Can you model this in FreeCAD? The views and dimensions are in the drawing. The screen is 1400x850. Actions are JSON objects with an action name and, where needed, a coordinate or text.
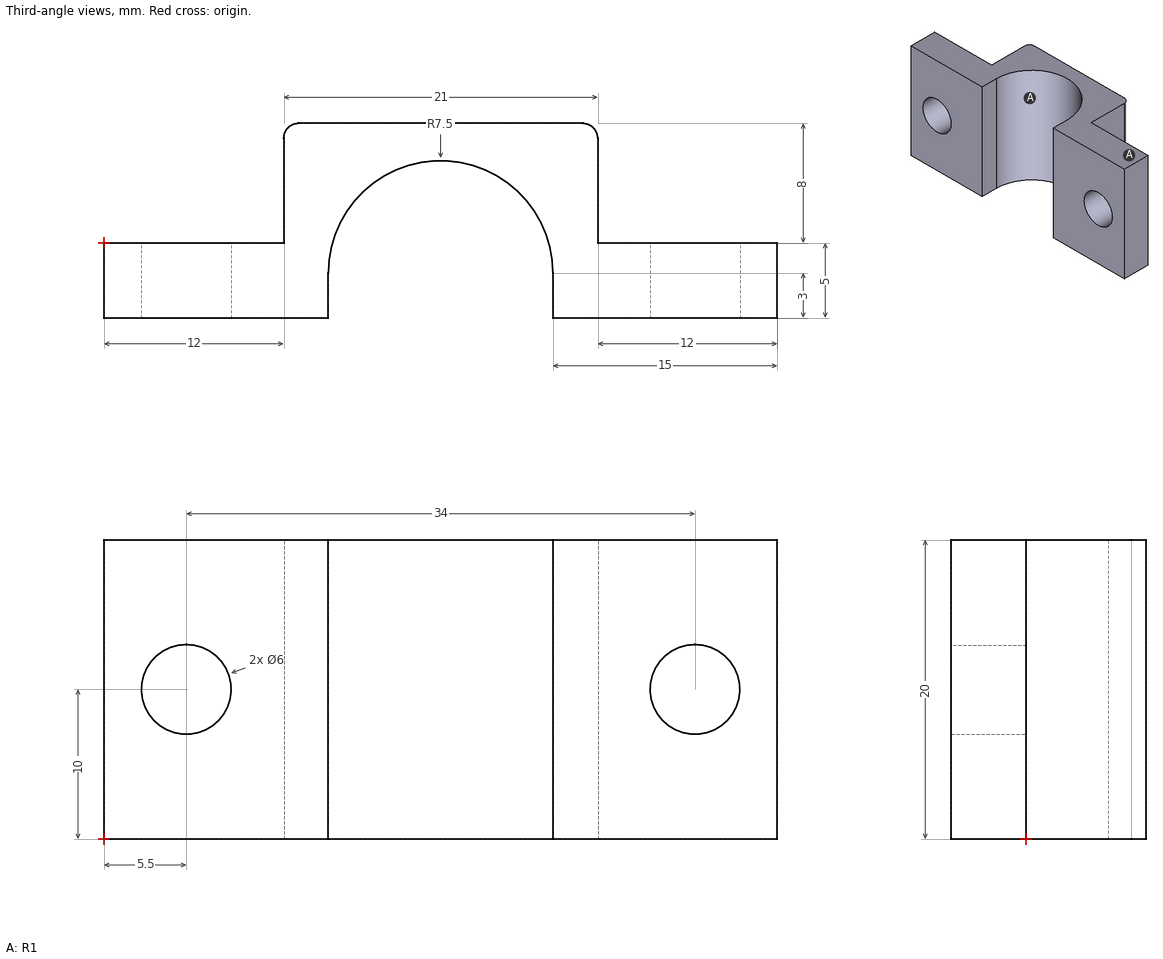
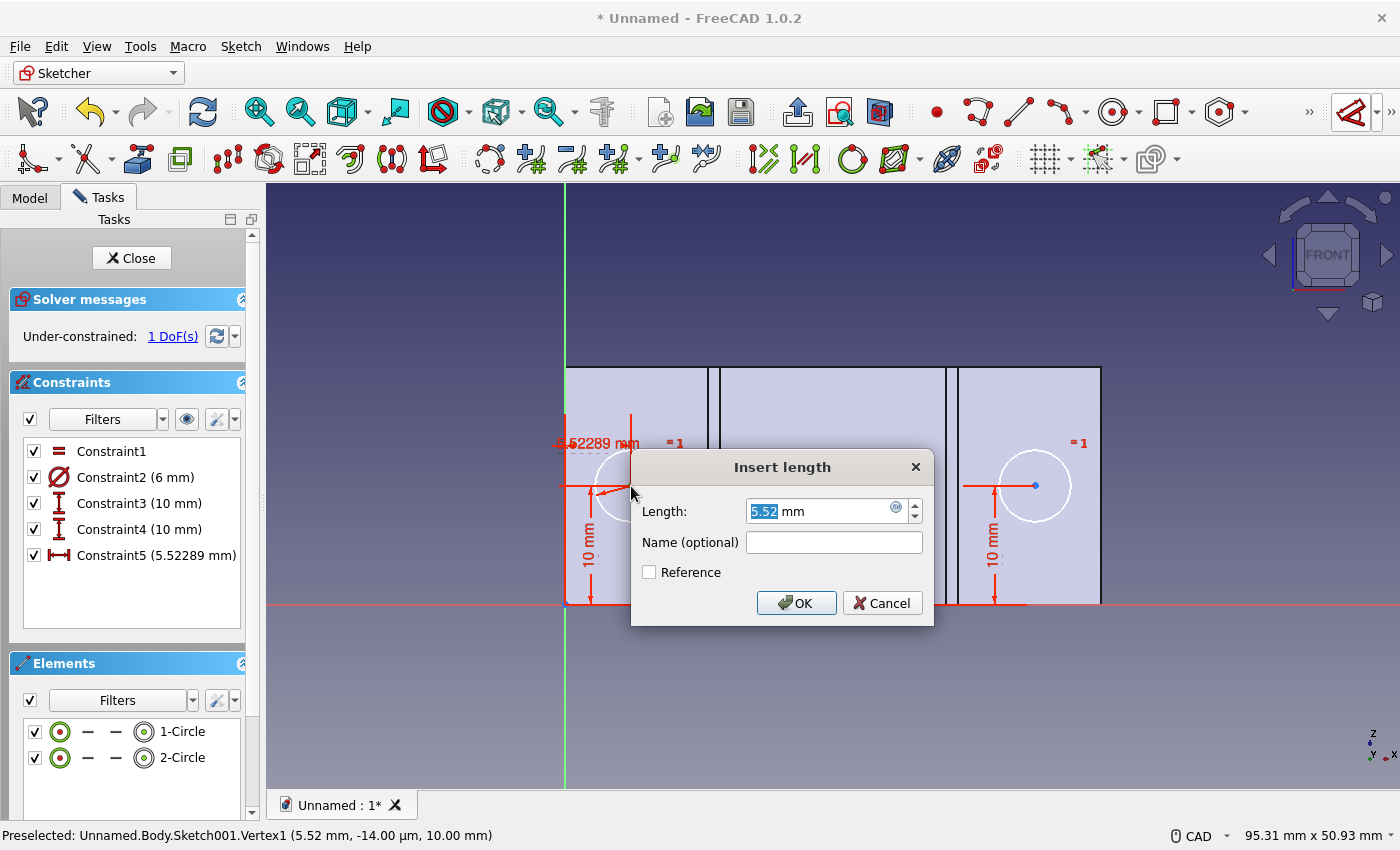
{"action": "type", "text": "5.5"}
{"action": "key", "text": "Return"}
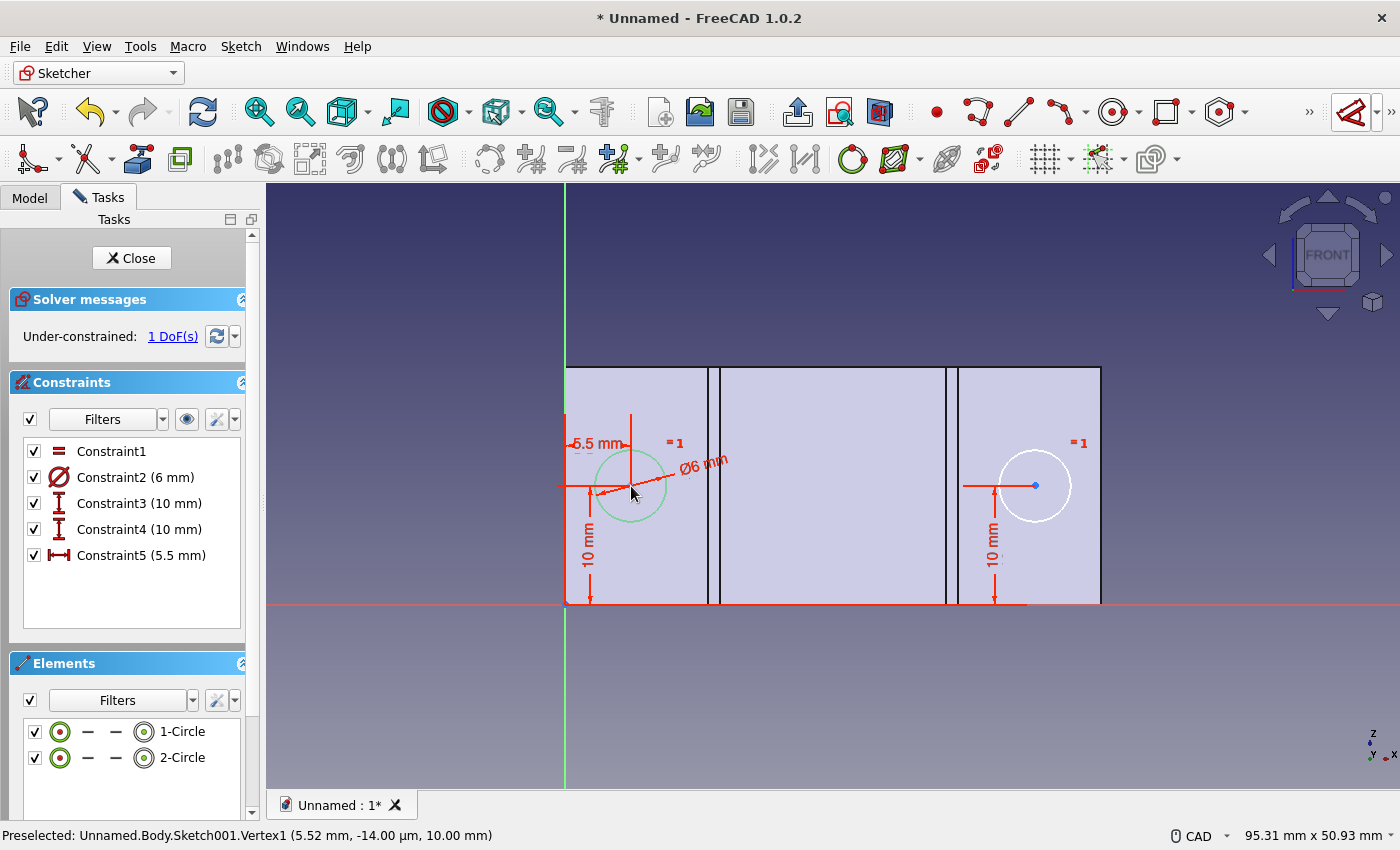
{"action": "left_click", "coordinate": [631, 486]}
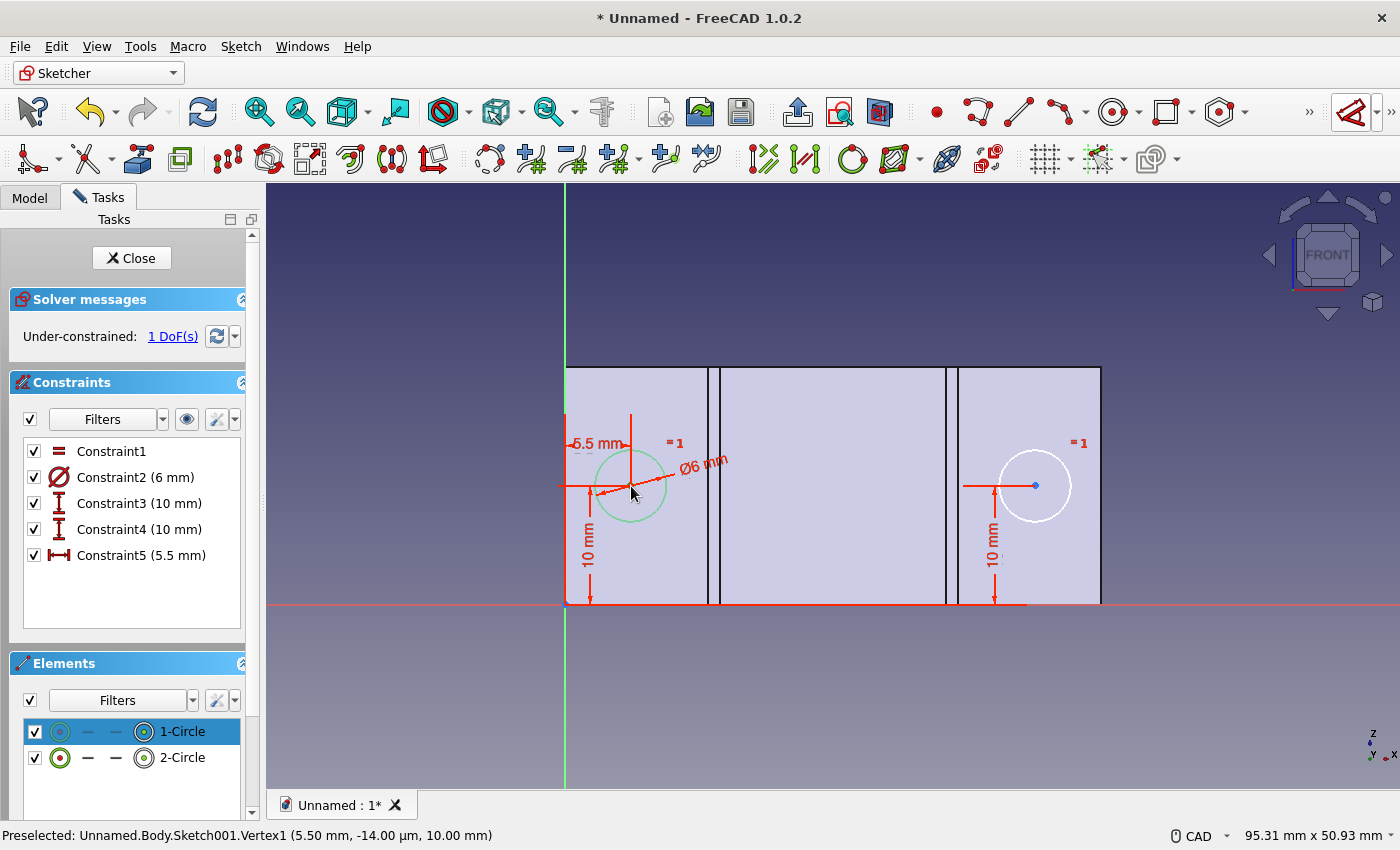
{"action": "left_click", "coordinate": [1035, 486]}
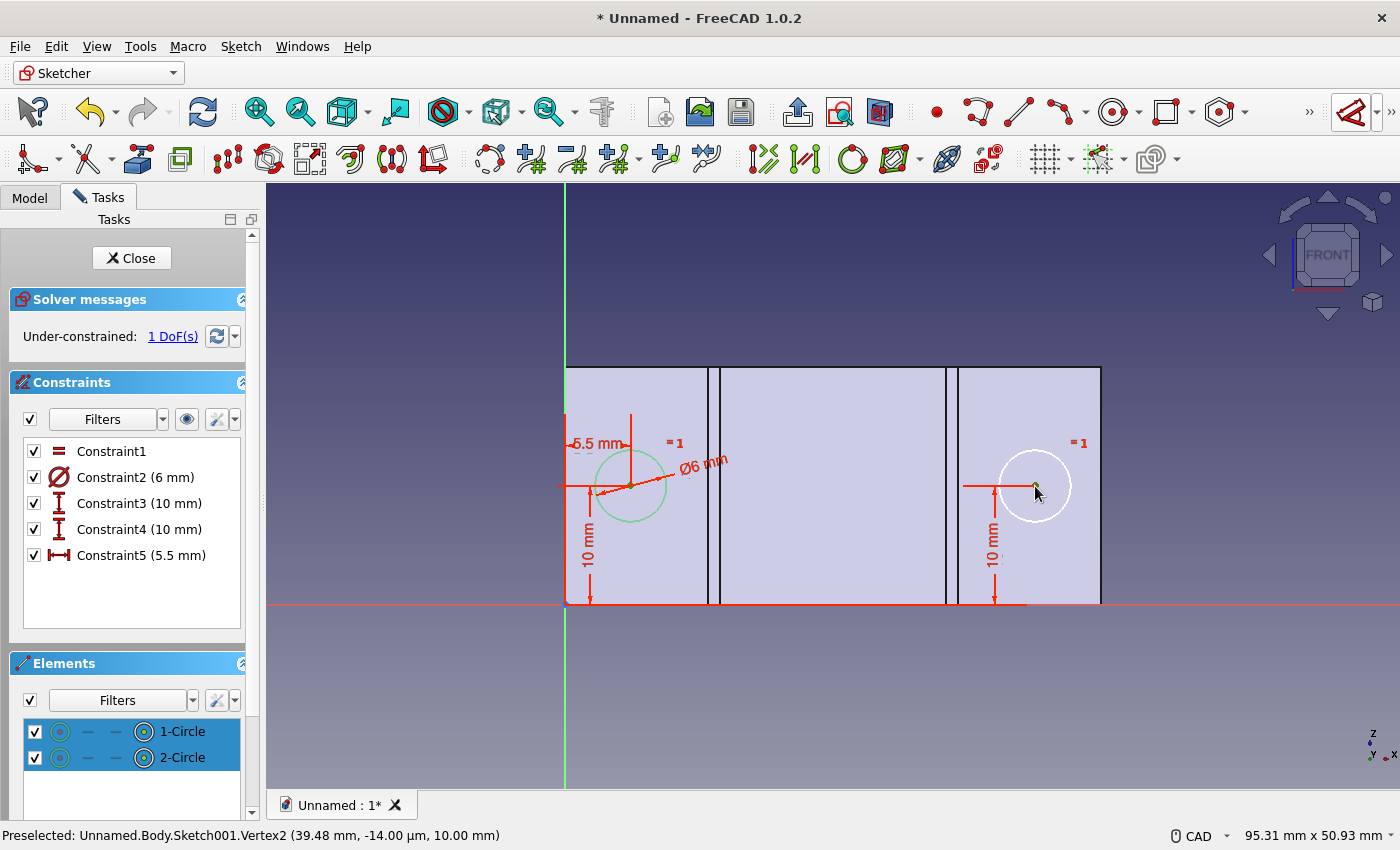
{"action": "key", "text": "l"}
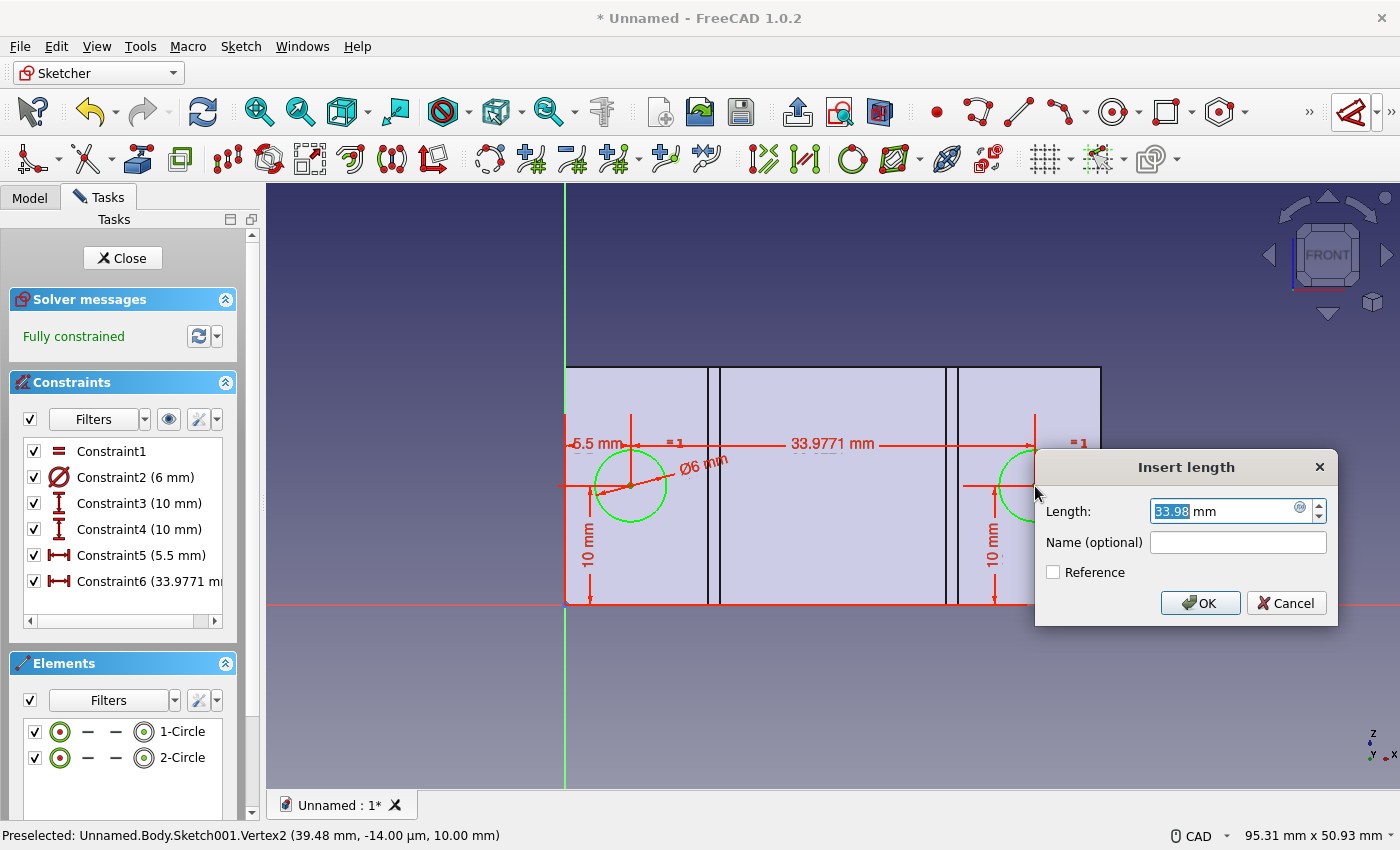
{"action": "type", "text": "34"}
{"action": "key", "text": "Return"}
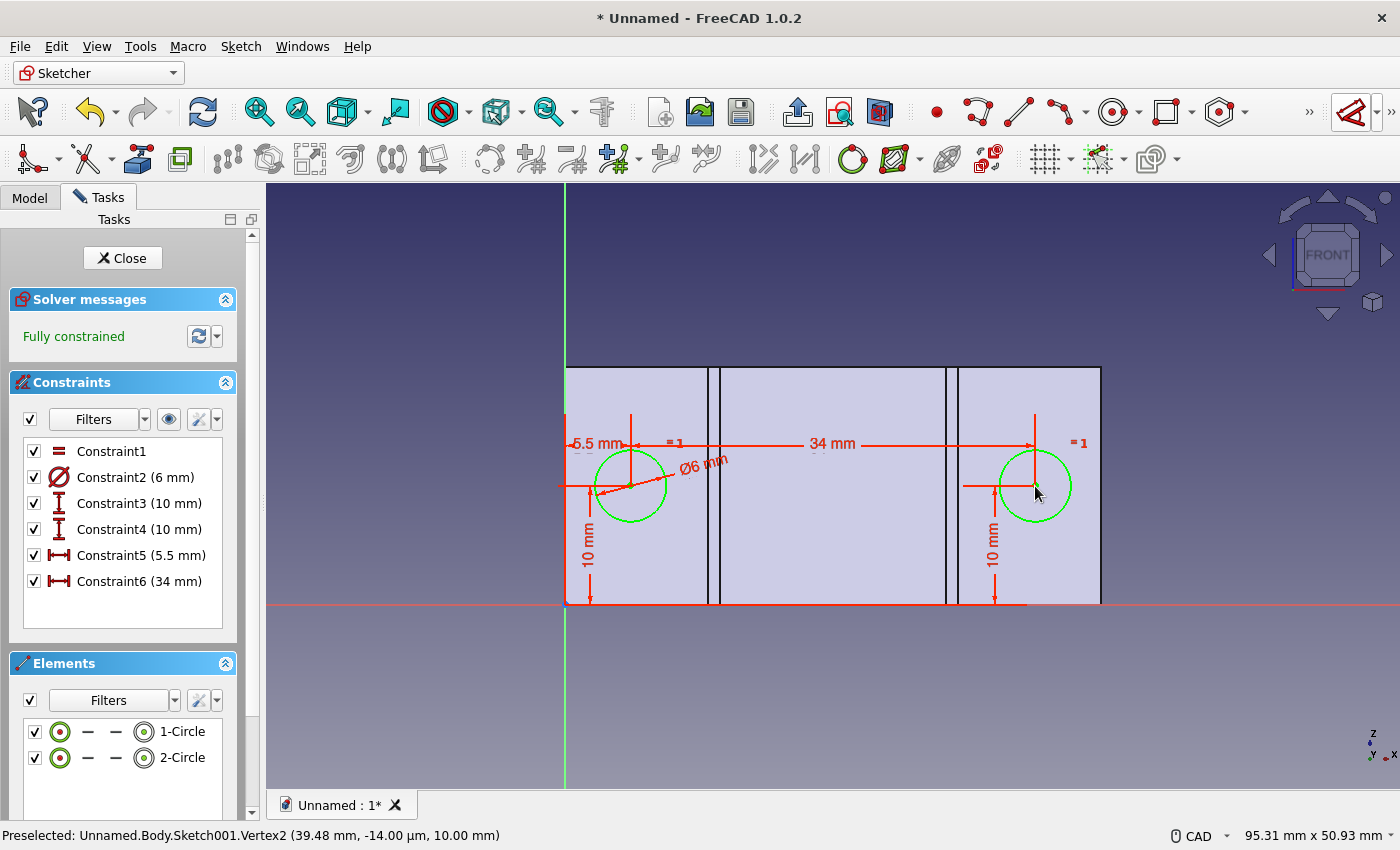
{"action": "left_click", "coordinate": [123, 258]}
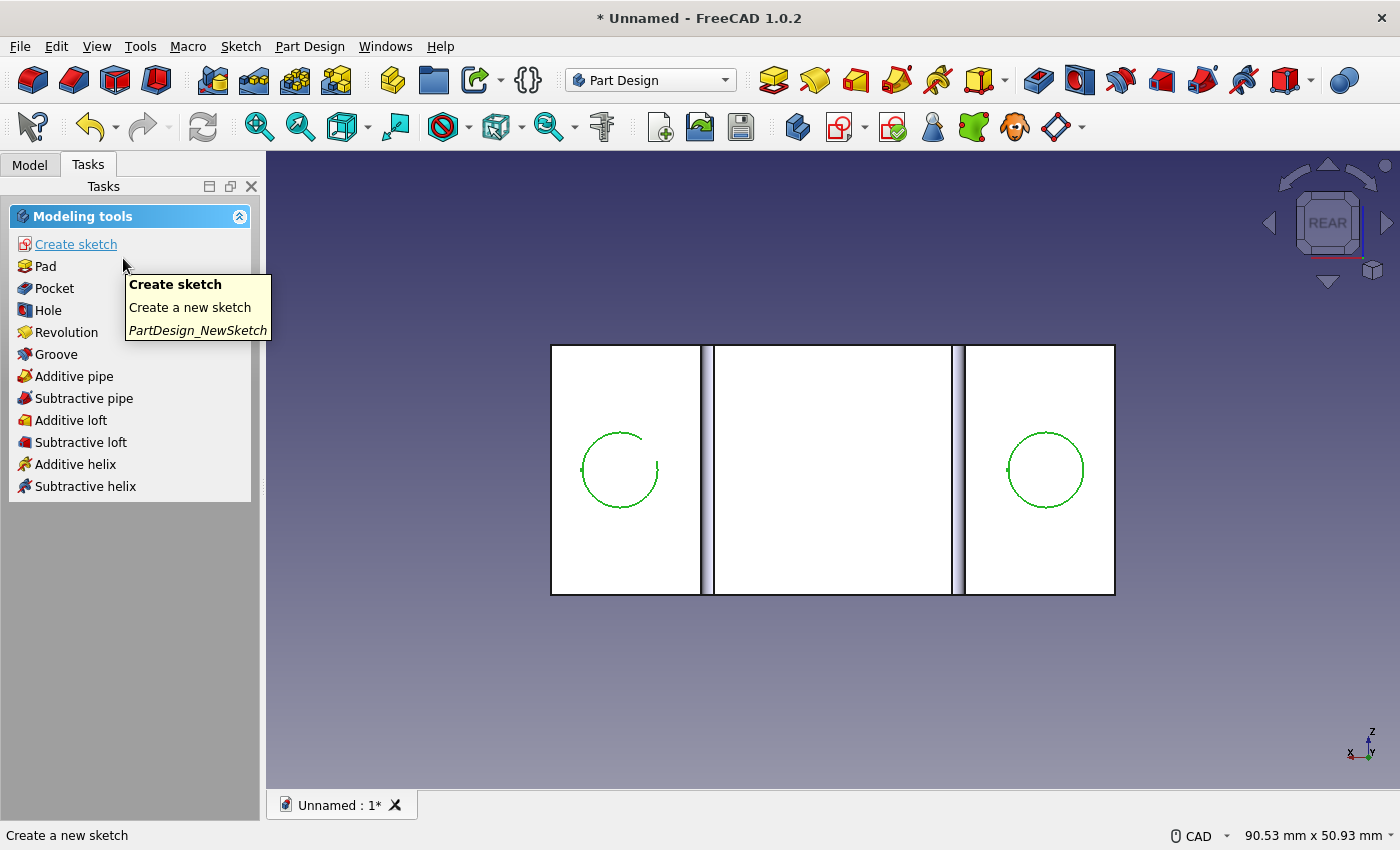
{"action": "left_click", "coordinate": [1039, 80]}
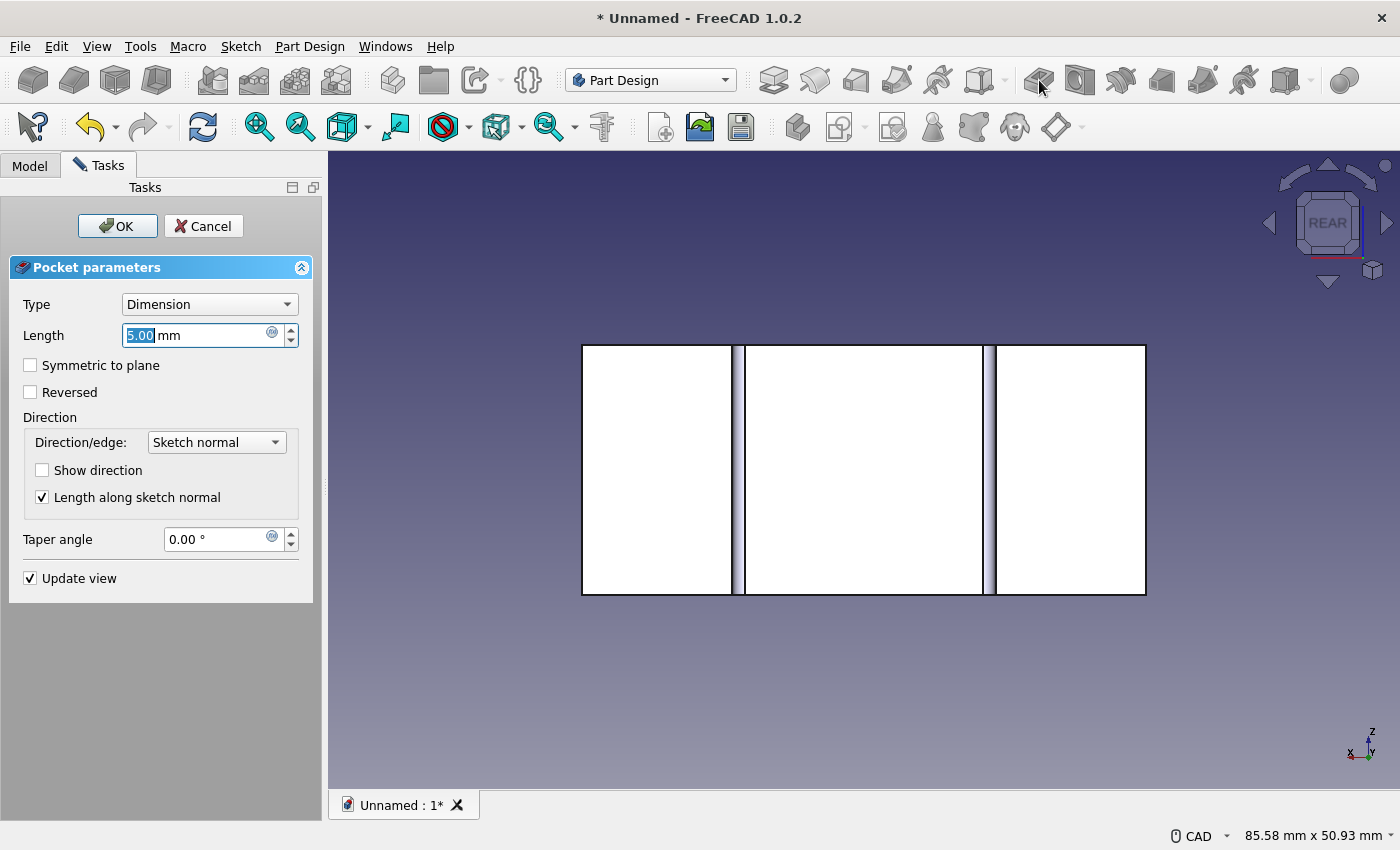
{"action": "left_click", "coordinate": [210, 304]}